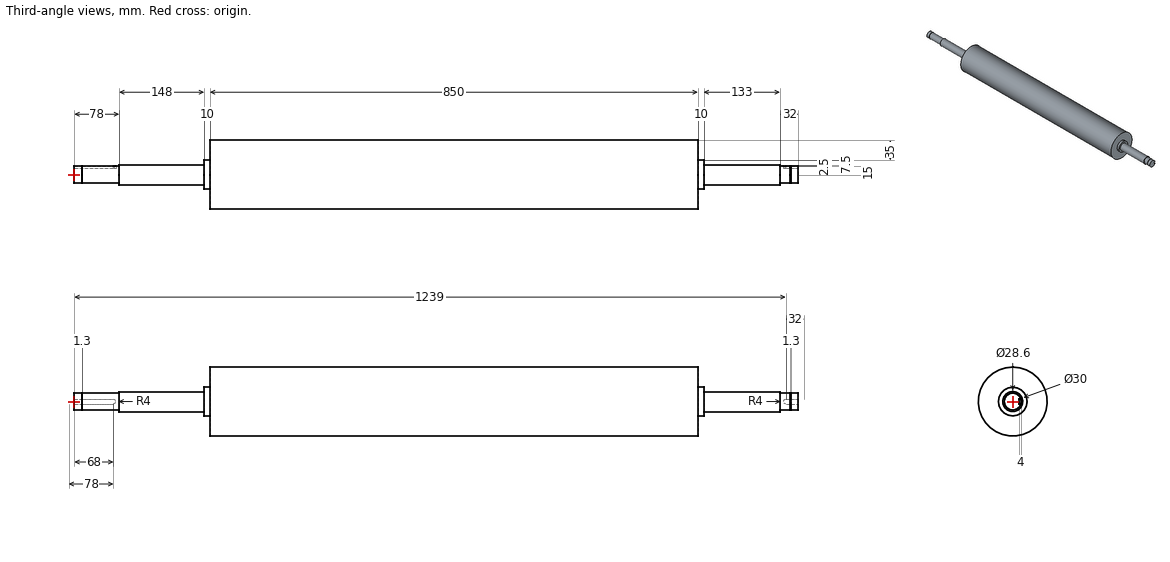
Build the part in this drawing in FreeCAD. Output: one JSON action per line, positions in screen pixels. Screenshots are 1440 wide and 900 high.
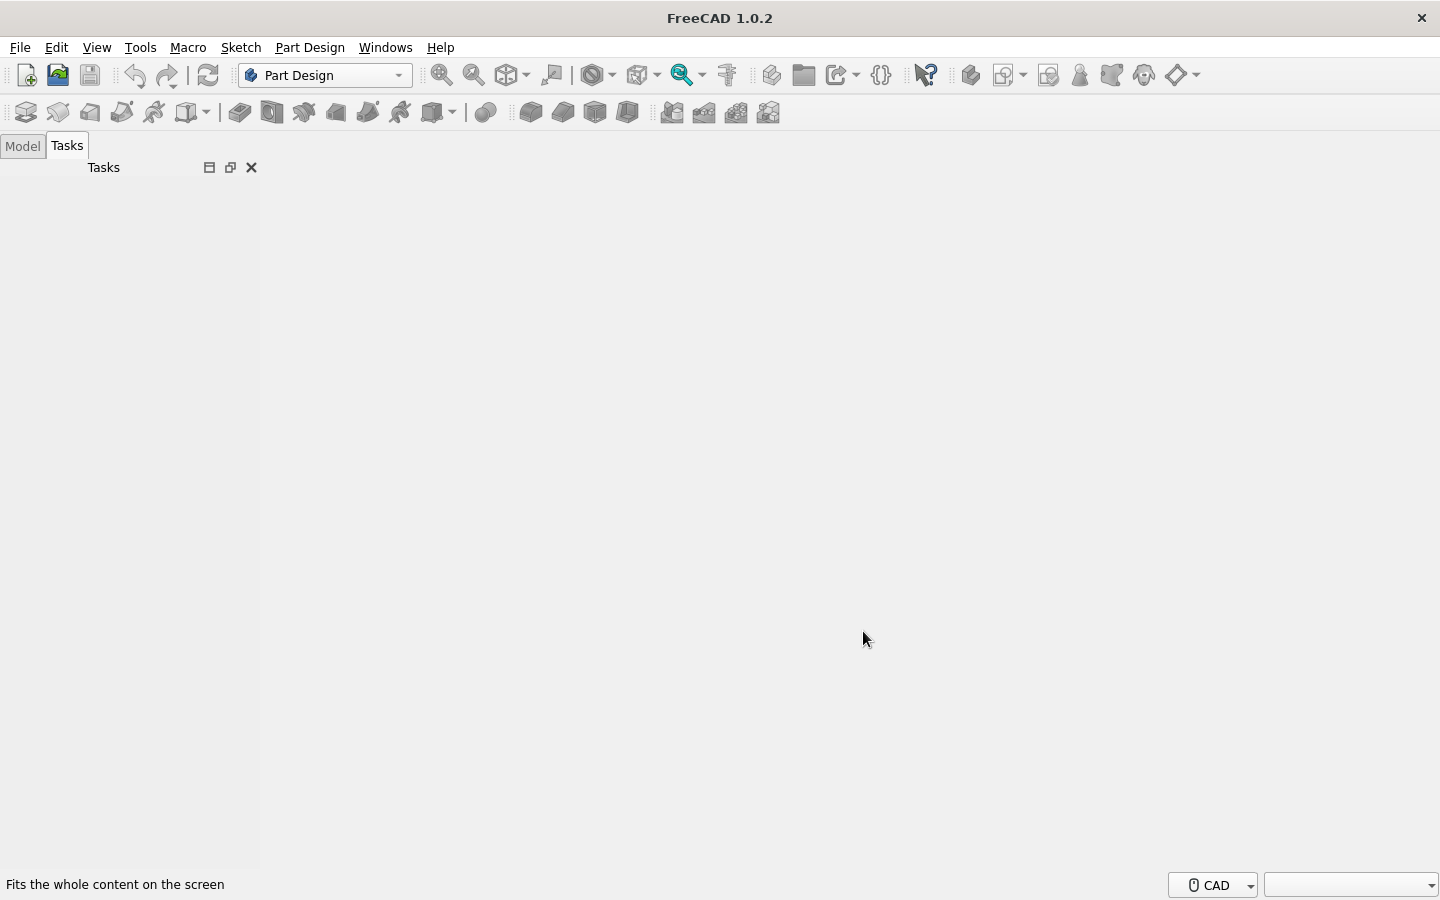
{"action": "key", "text": "ctrl+n"}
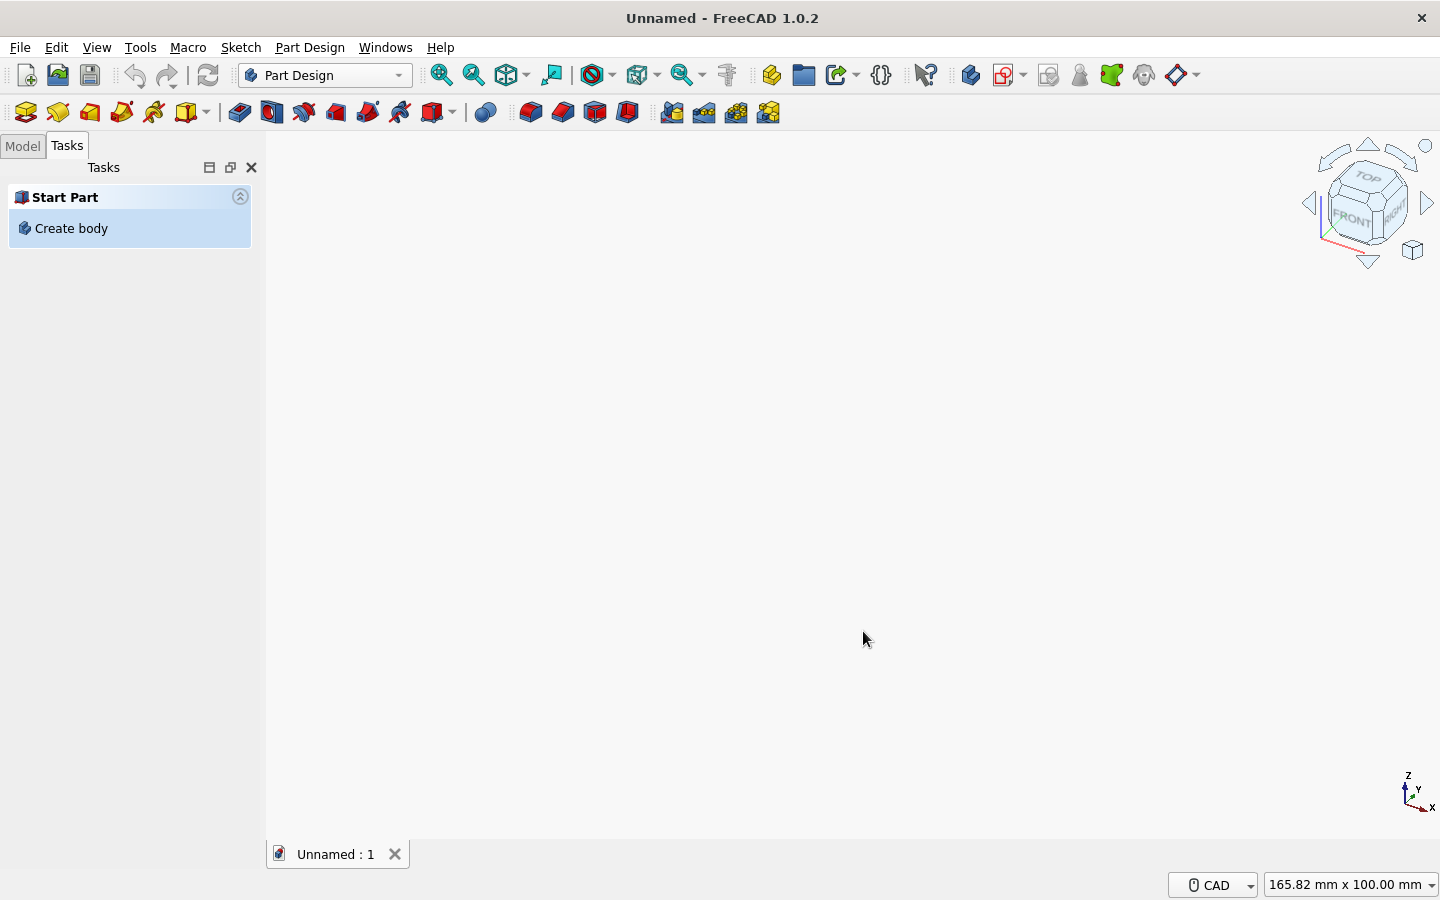
{"action": "left_click", "coordinate": [1004, 76]}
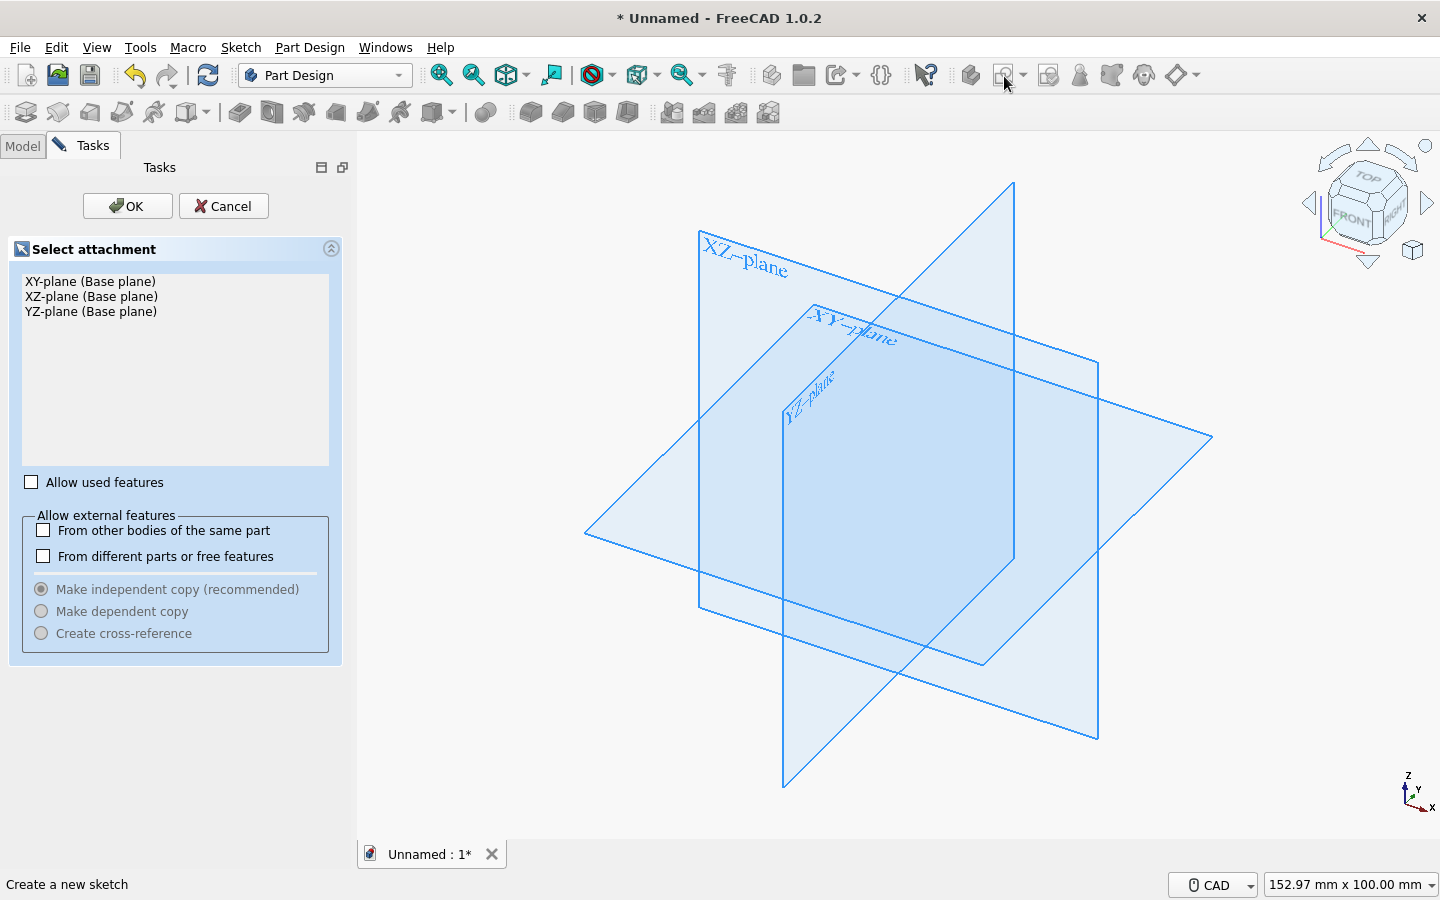
{"action": "left_click", "coordinate": [82, 282]}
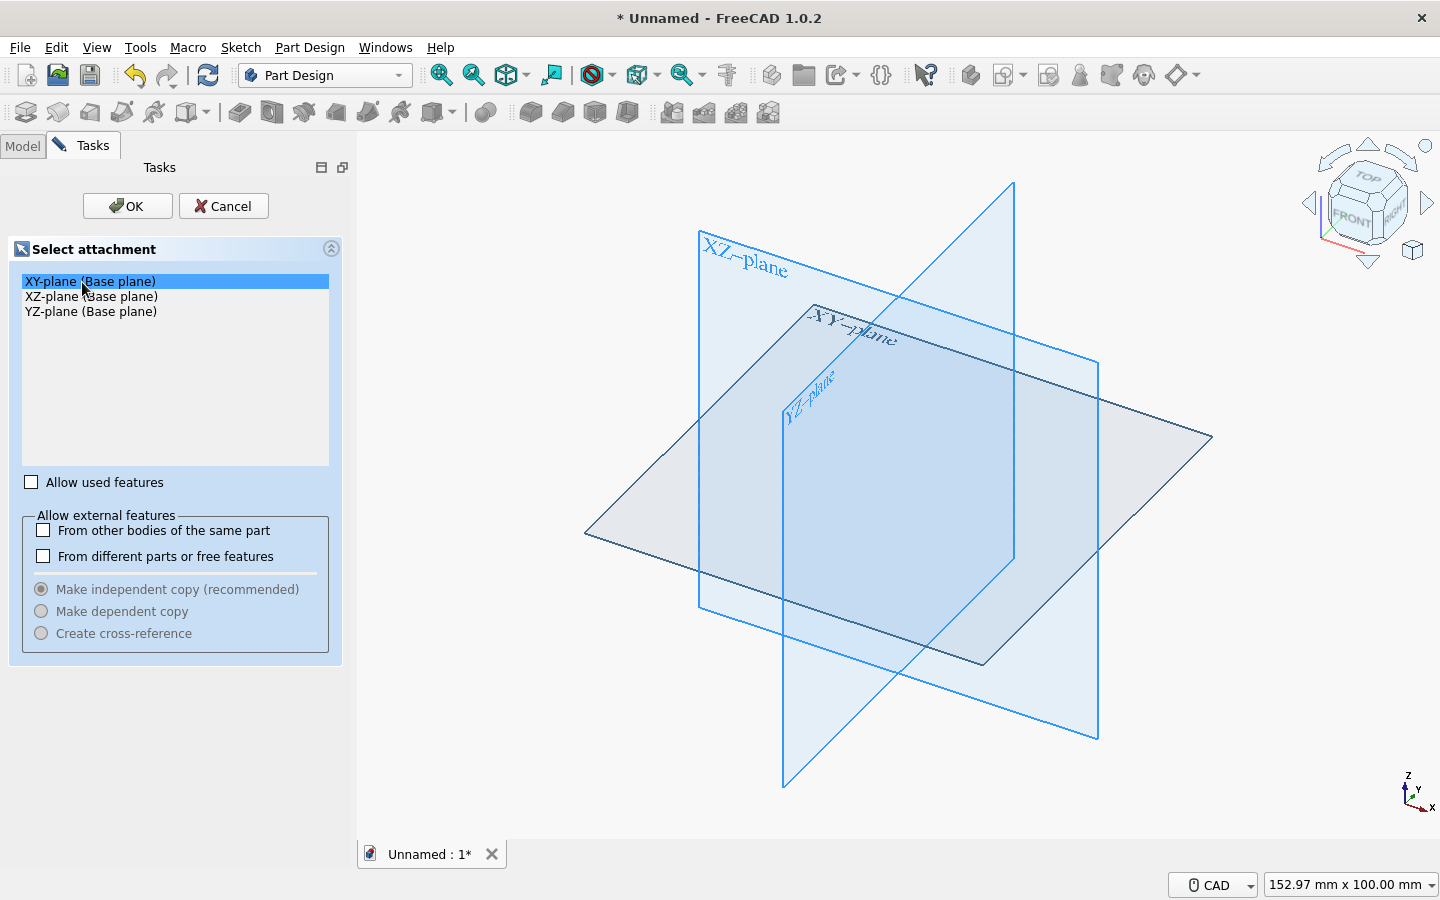
{"action": "left_click", "coordinate": [128, 206]}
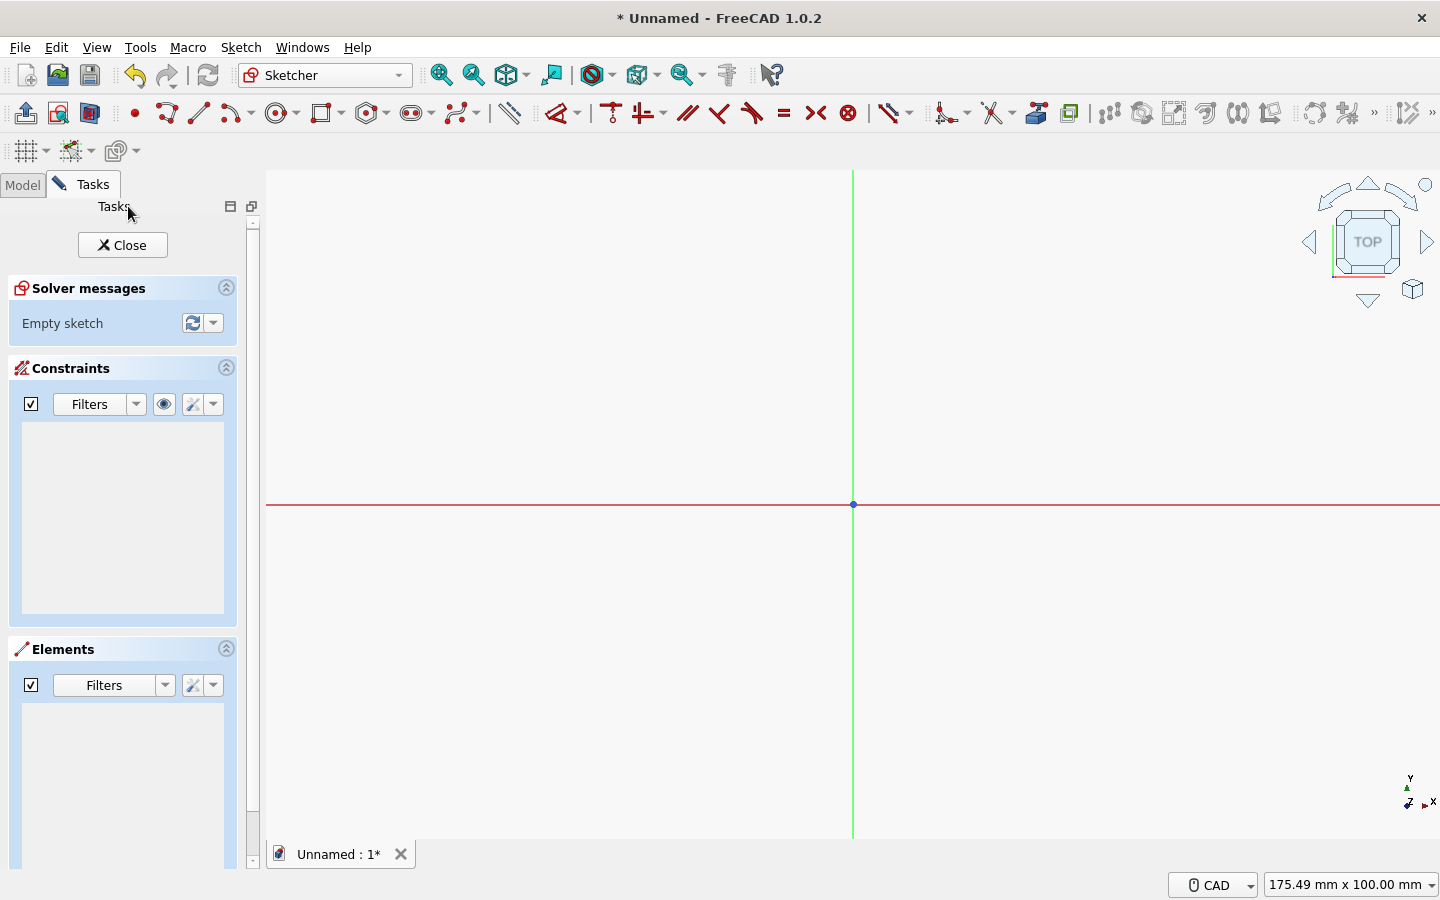
{"action": "scroll", "coordinate": [441, 521], "scroll_direction": "down", "scroll_amount": 13}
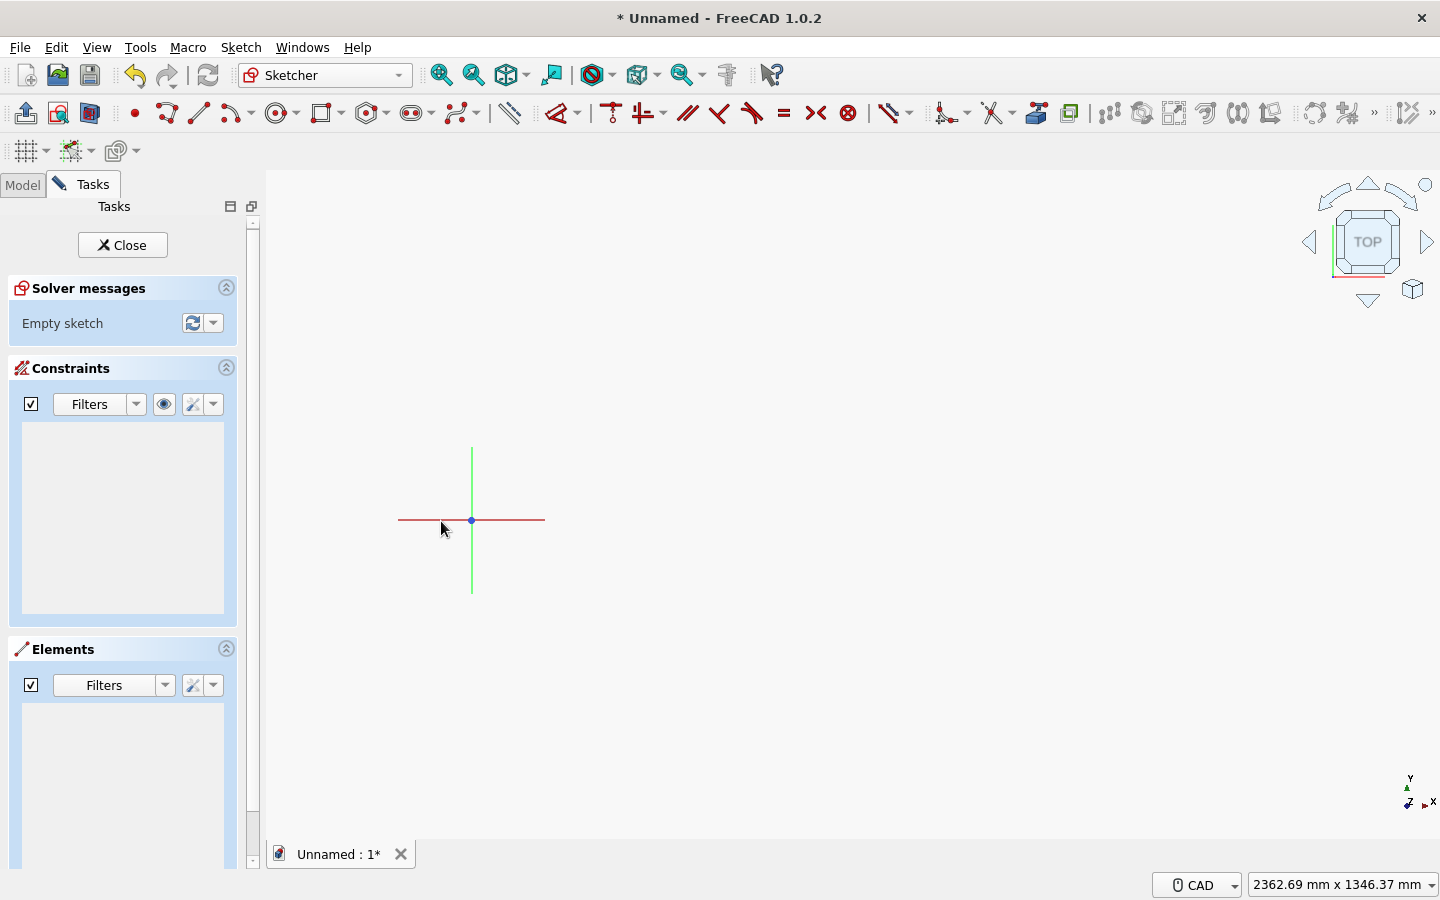
{"action": "key", "text": "g m"}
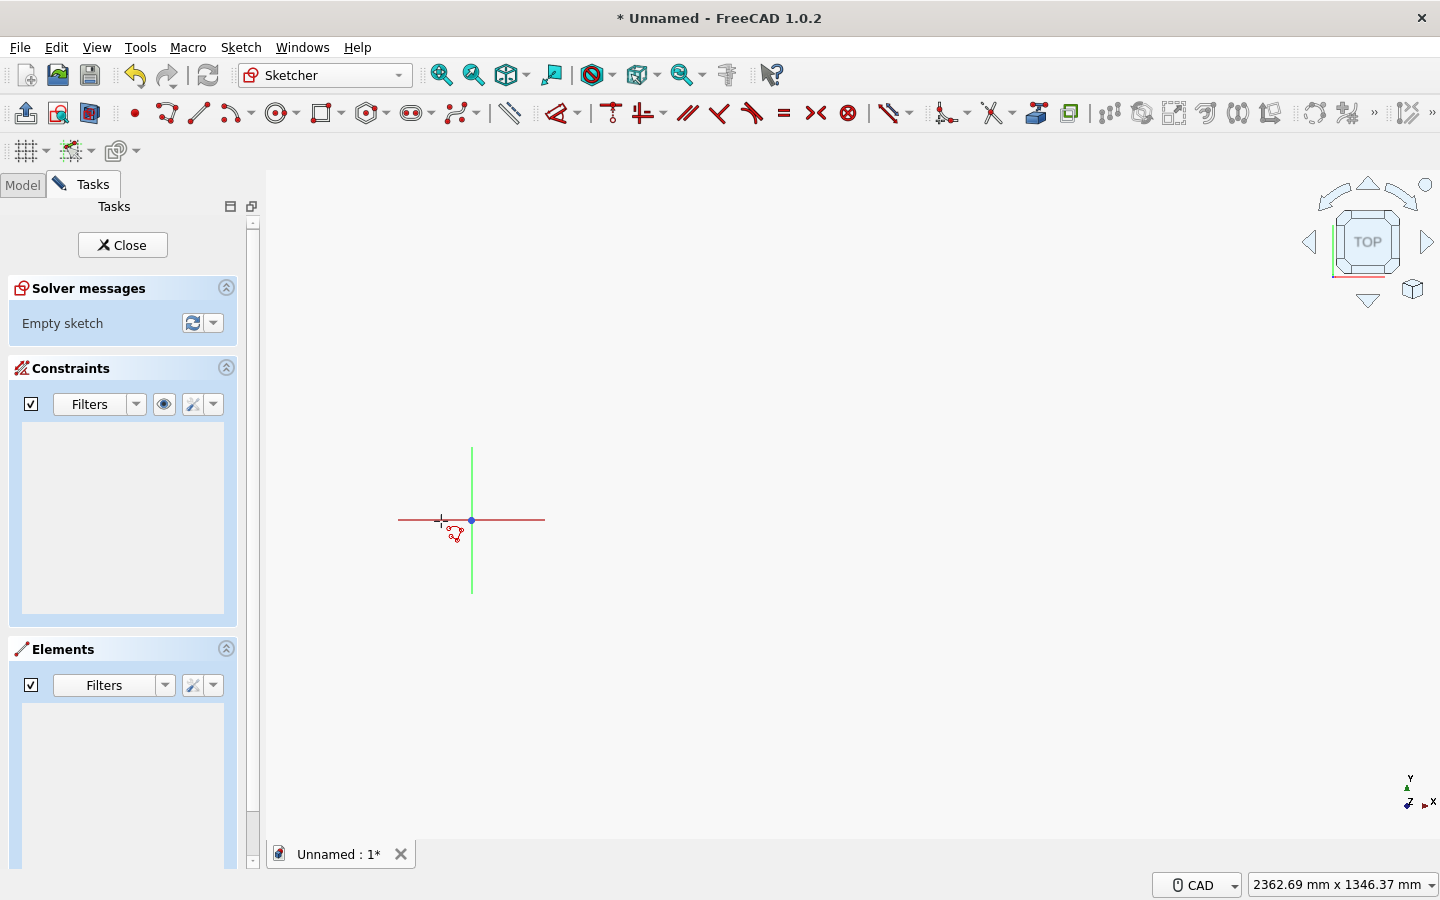
{"action": "left_click", "coordinate": [472, 520]}
{"action": "left_click", "coordinate": [1098, 511]}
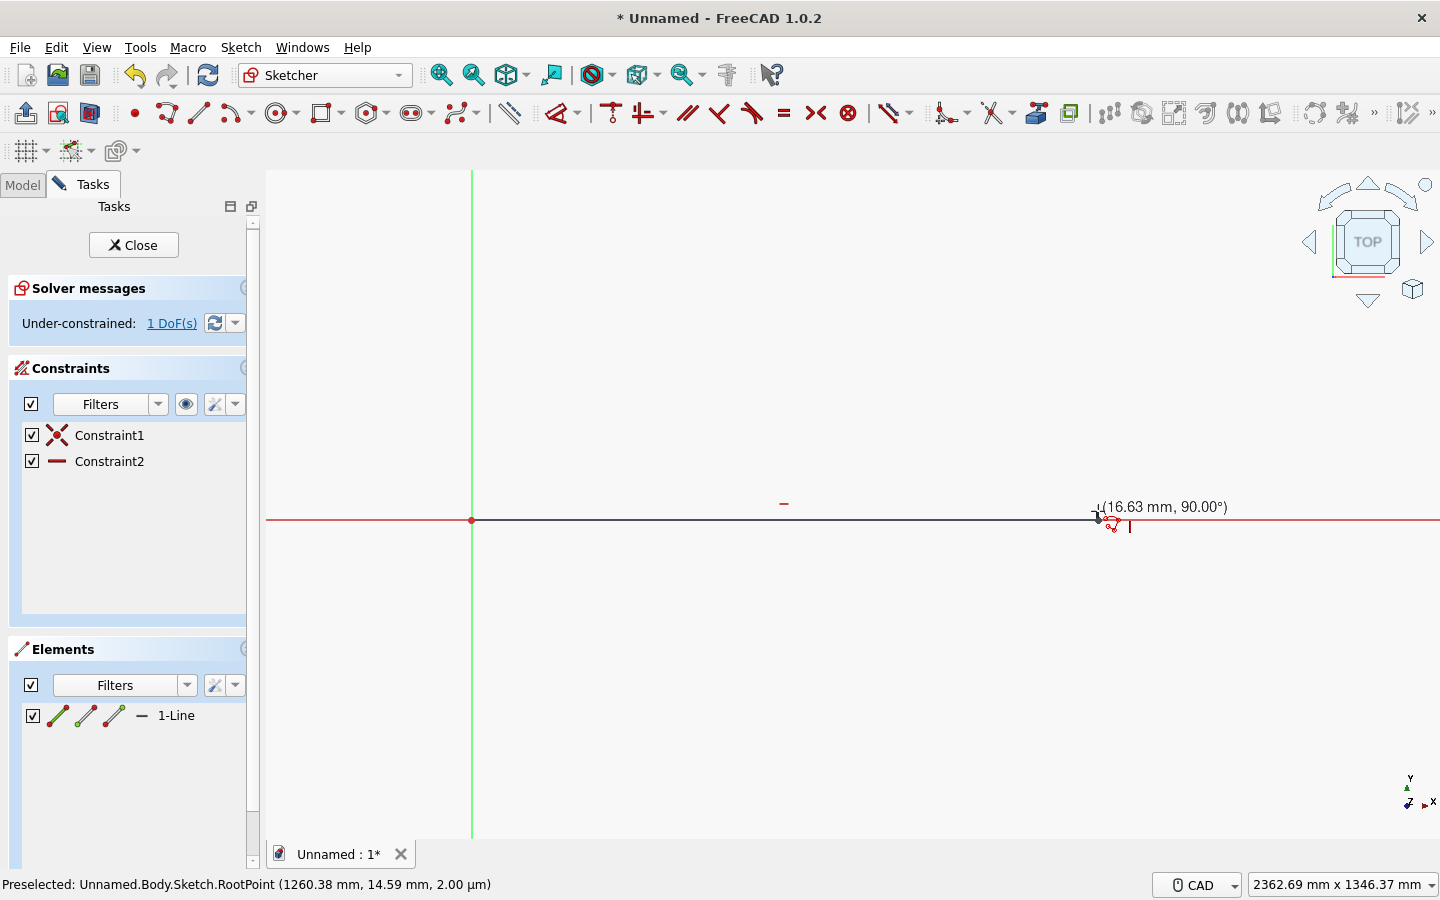
{"action": "scroll", "coordinate": [1098, 513], "scroll_direction": "up", "scroll_amount": 4}